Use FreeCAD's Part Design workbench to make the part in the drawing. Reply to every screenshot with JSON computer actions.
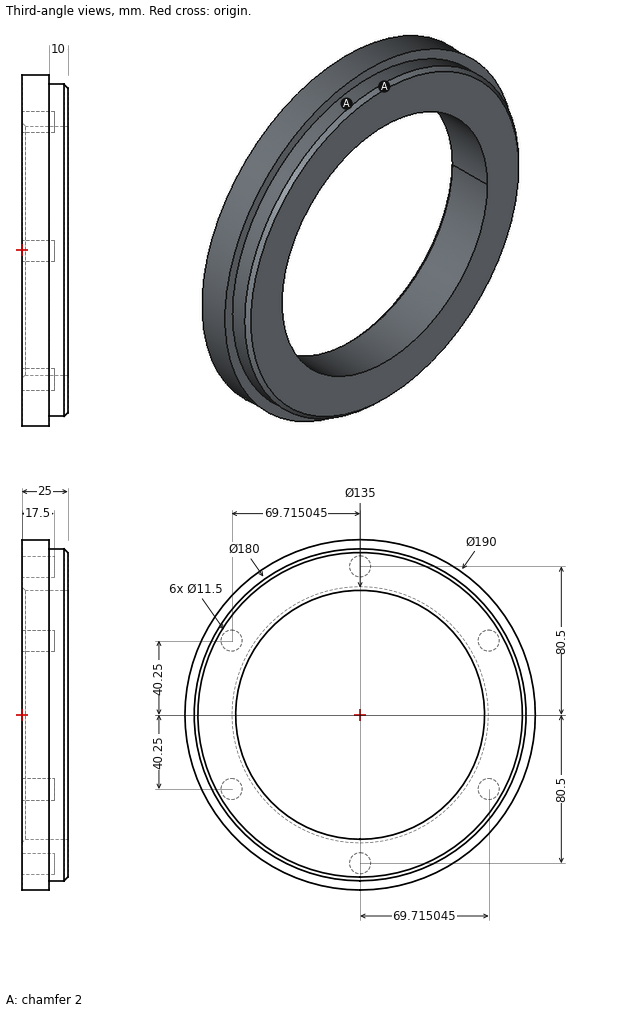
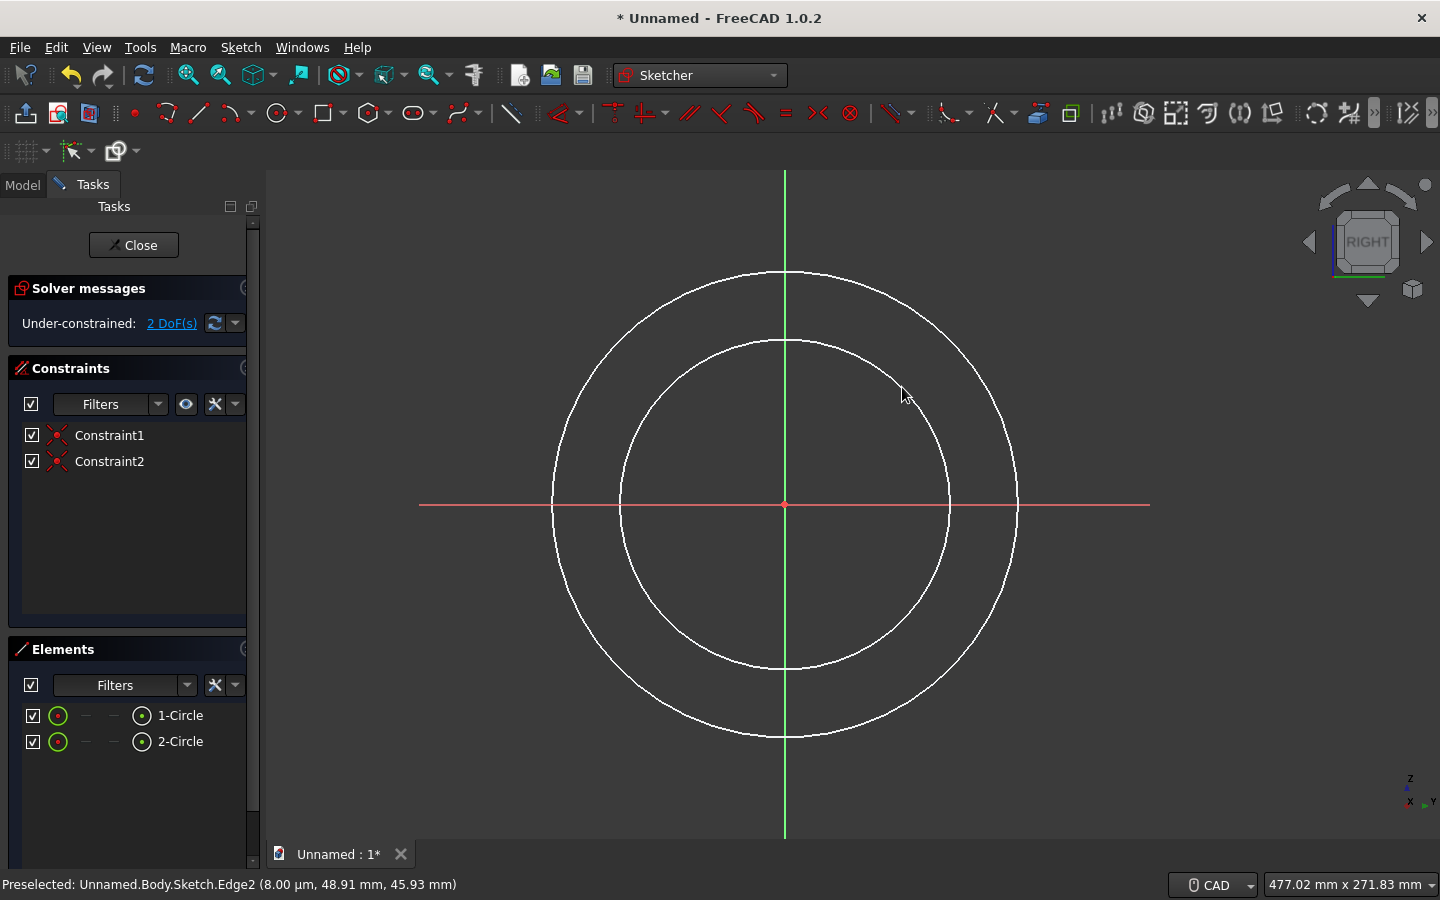
{"action": "left_click", "coordinate": [558, 114]}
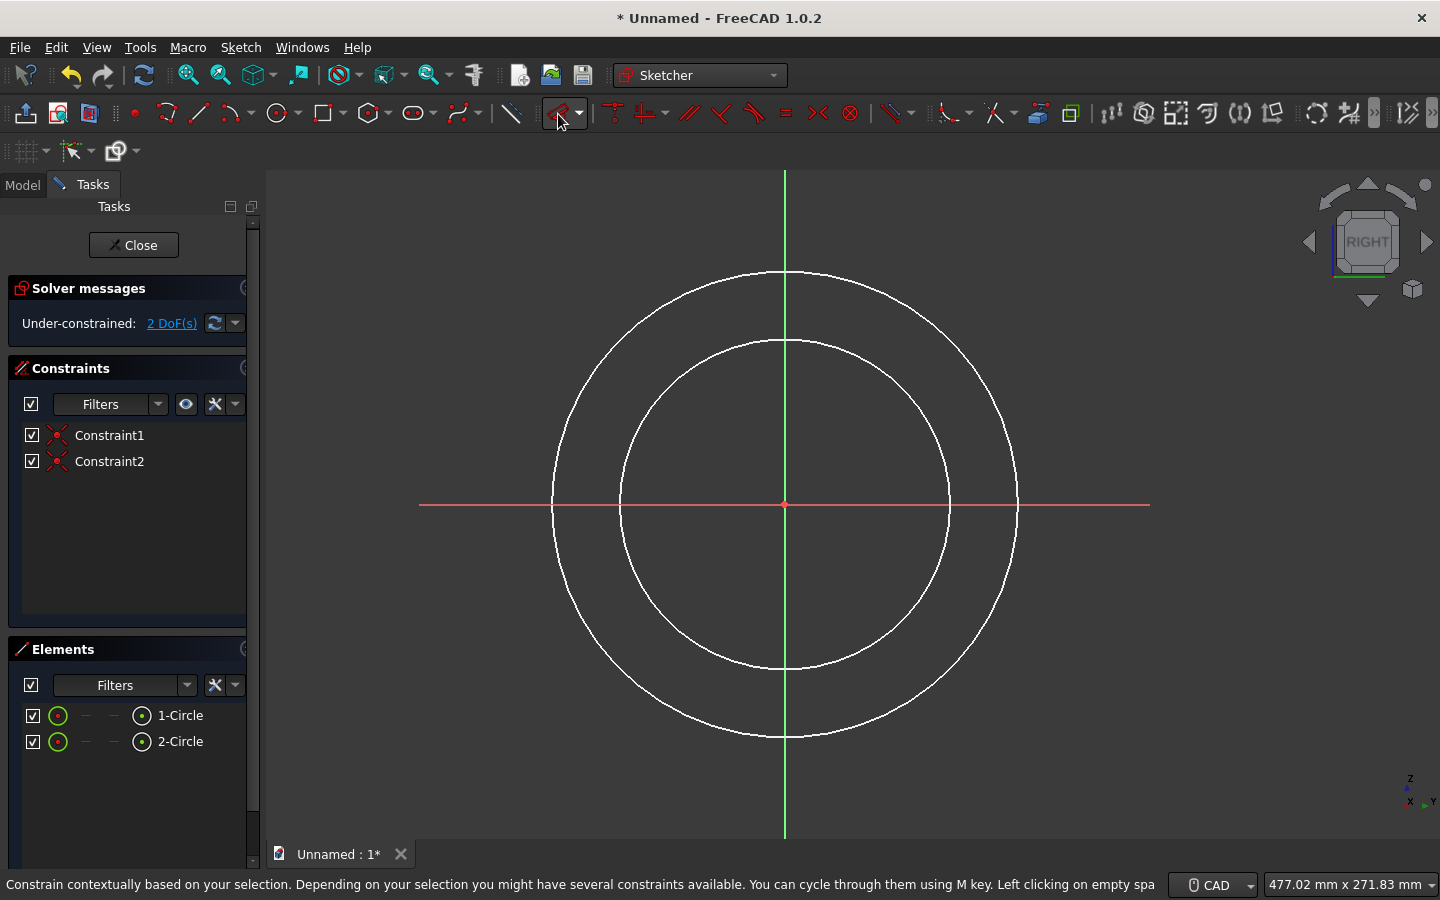
{"action": "left_click", "coordinate": [949, 339]}
{"action": "left_click", "coordinate": [972, 316]}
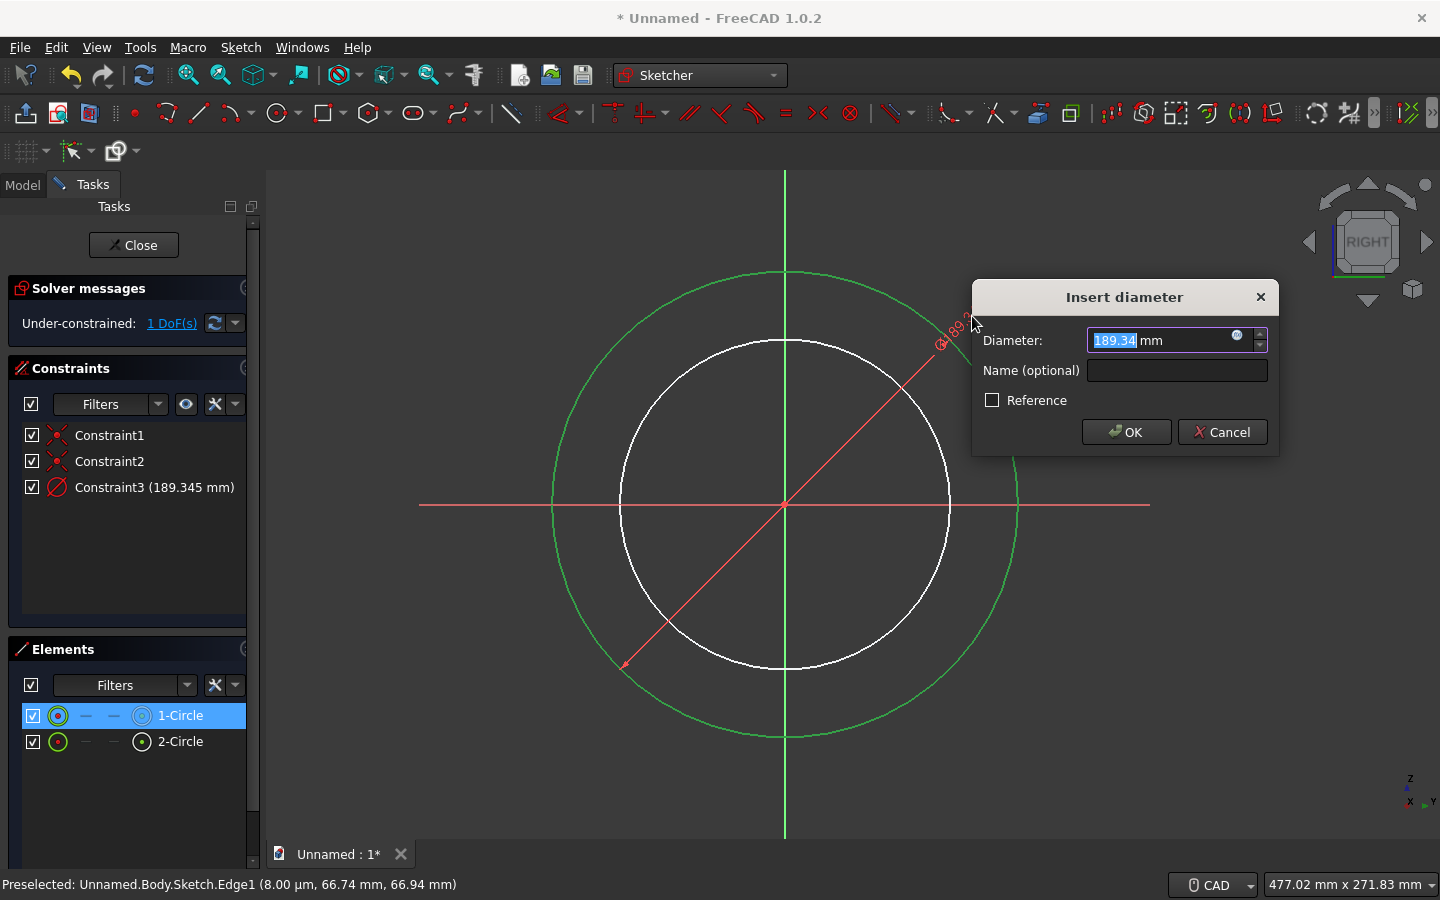
{"action": "type", "text": "190"}
{"action": "key", "text": "Return"}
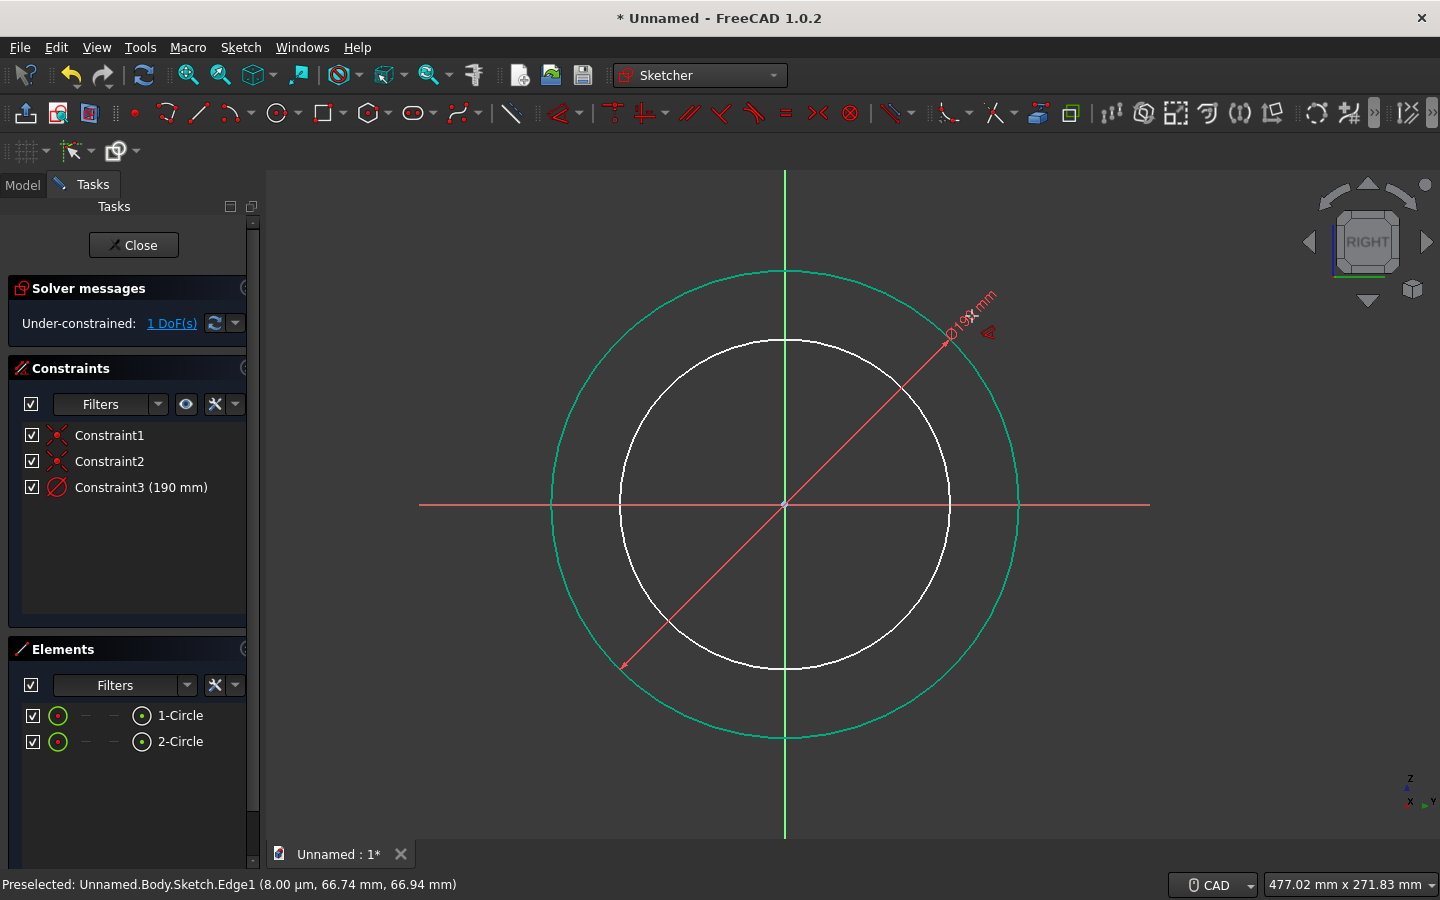
{"action": "left_click", "coordinate": [901, 387]}
{"action": "left_click", "coordinate": [923, 364]}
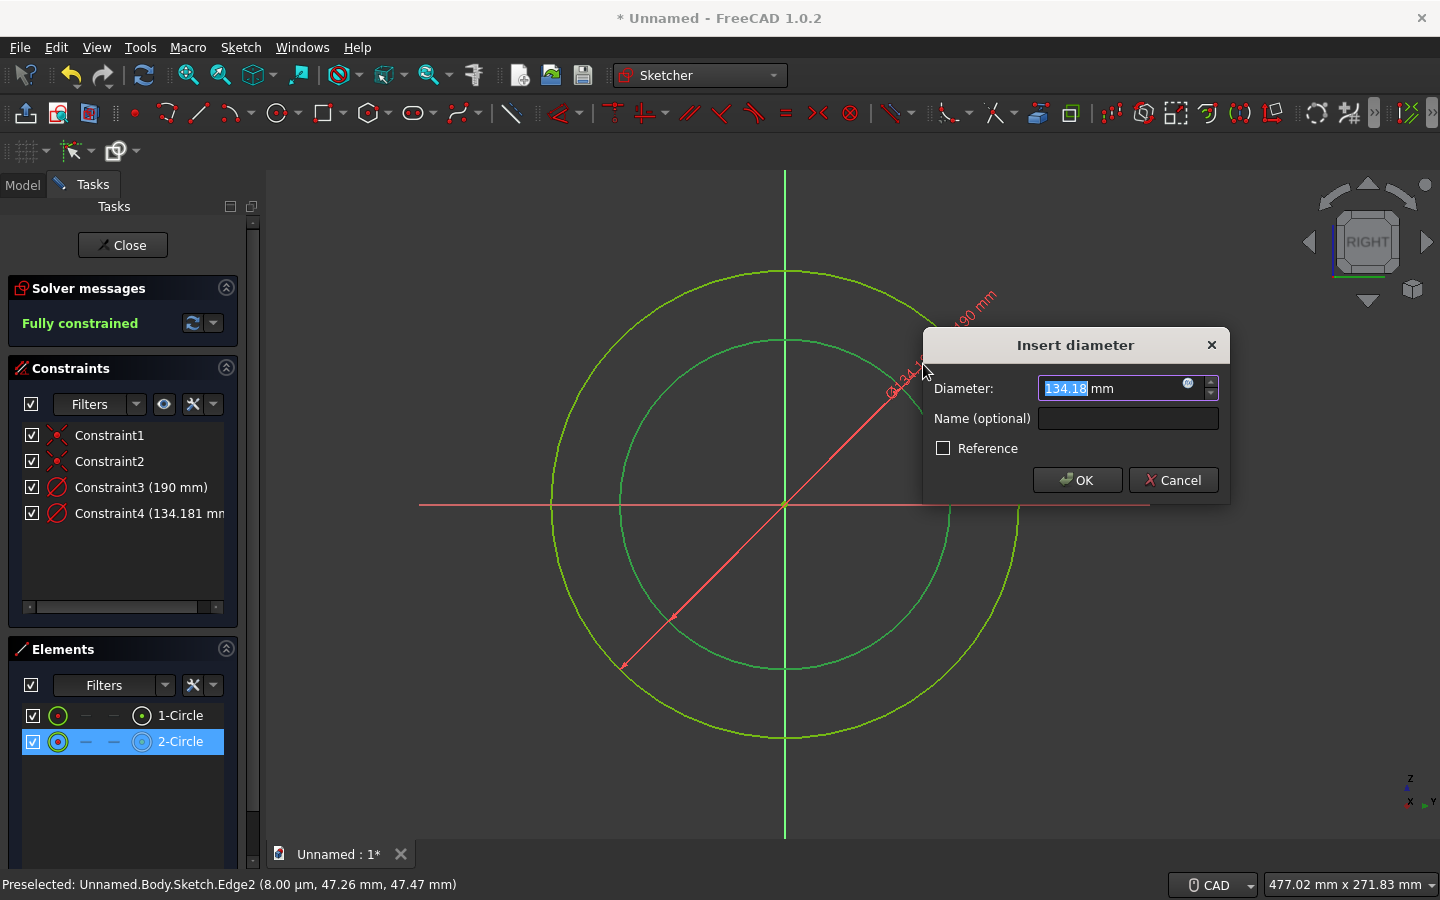
{"action": "type", "text": "135"}
{"action": "key", "text": "Return"}
{"action": "key", "text": "Escape"}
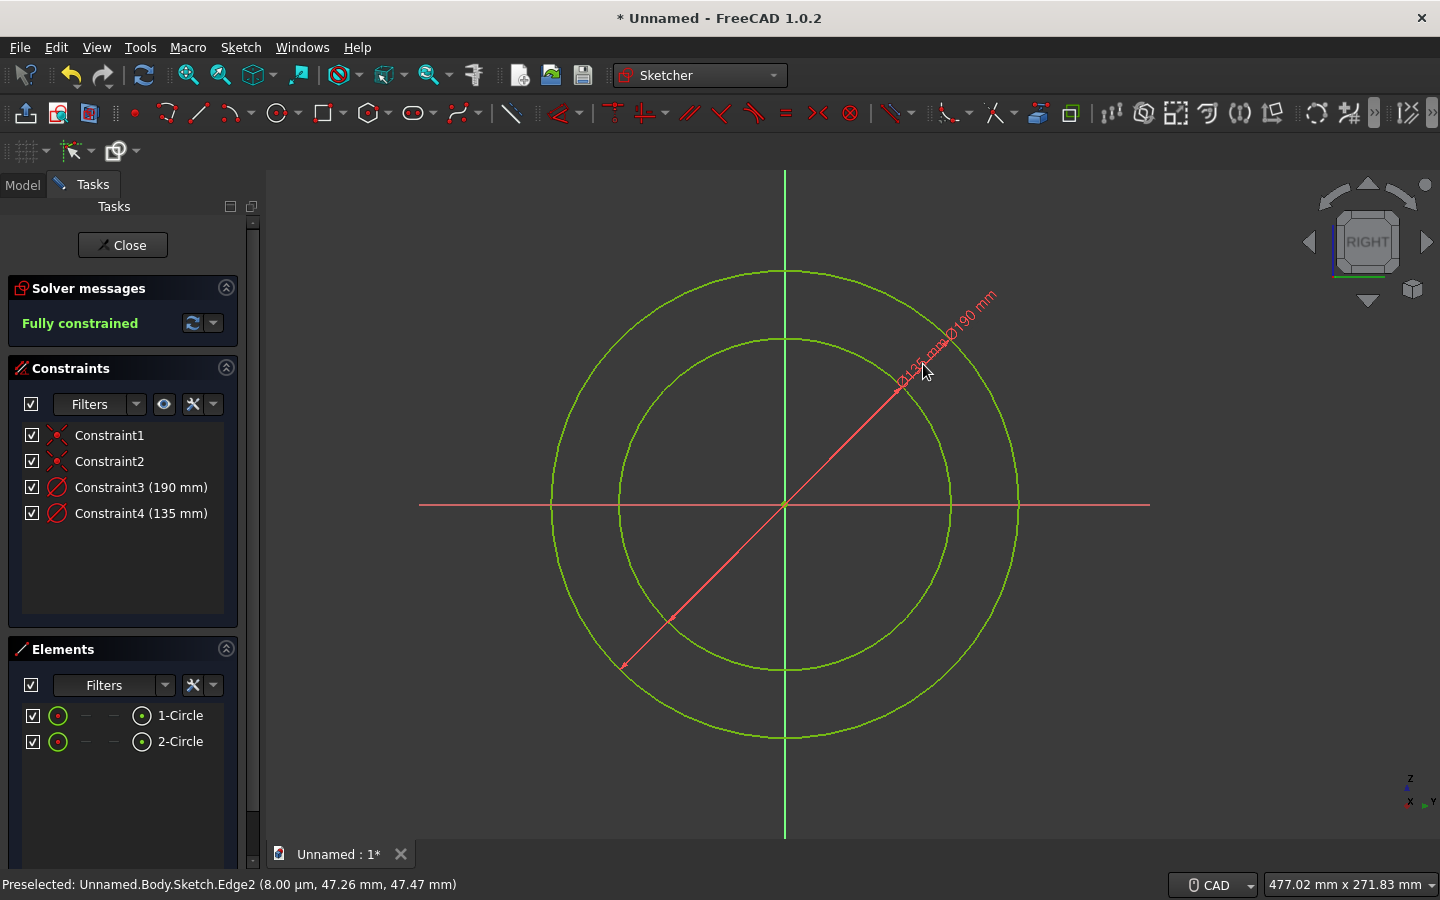
{"action": "left_click", "coordinate": [123, 245]}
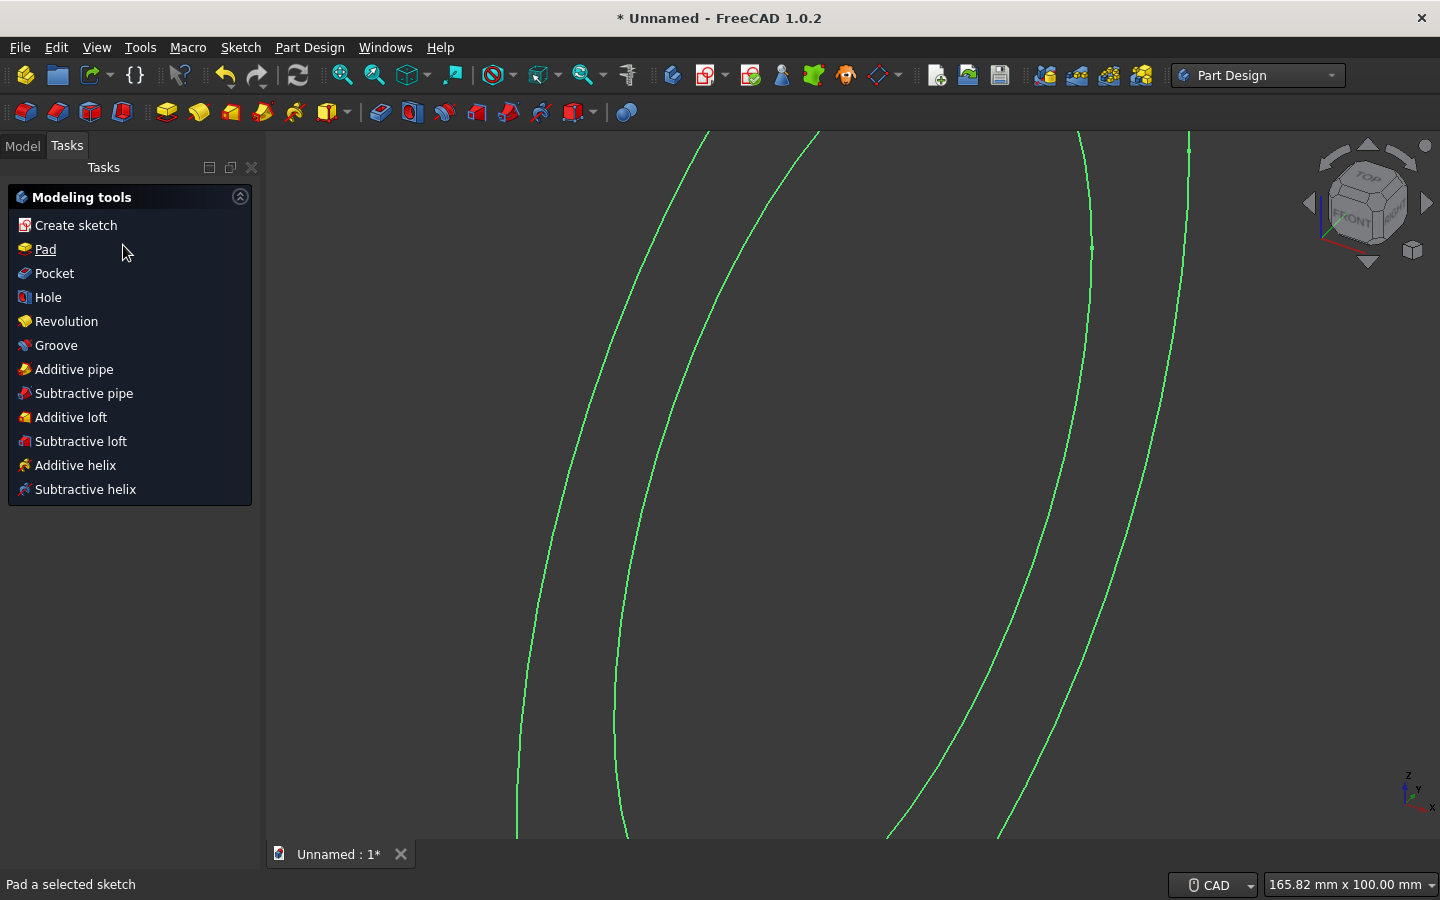
{"action": "left_click", "coordinate": [168, 112]}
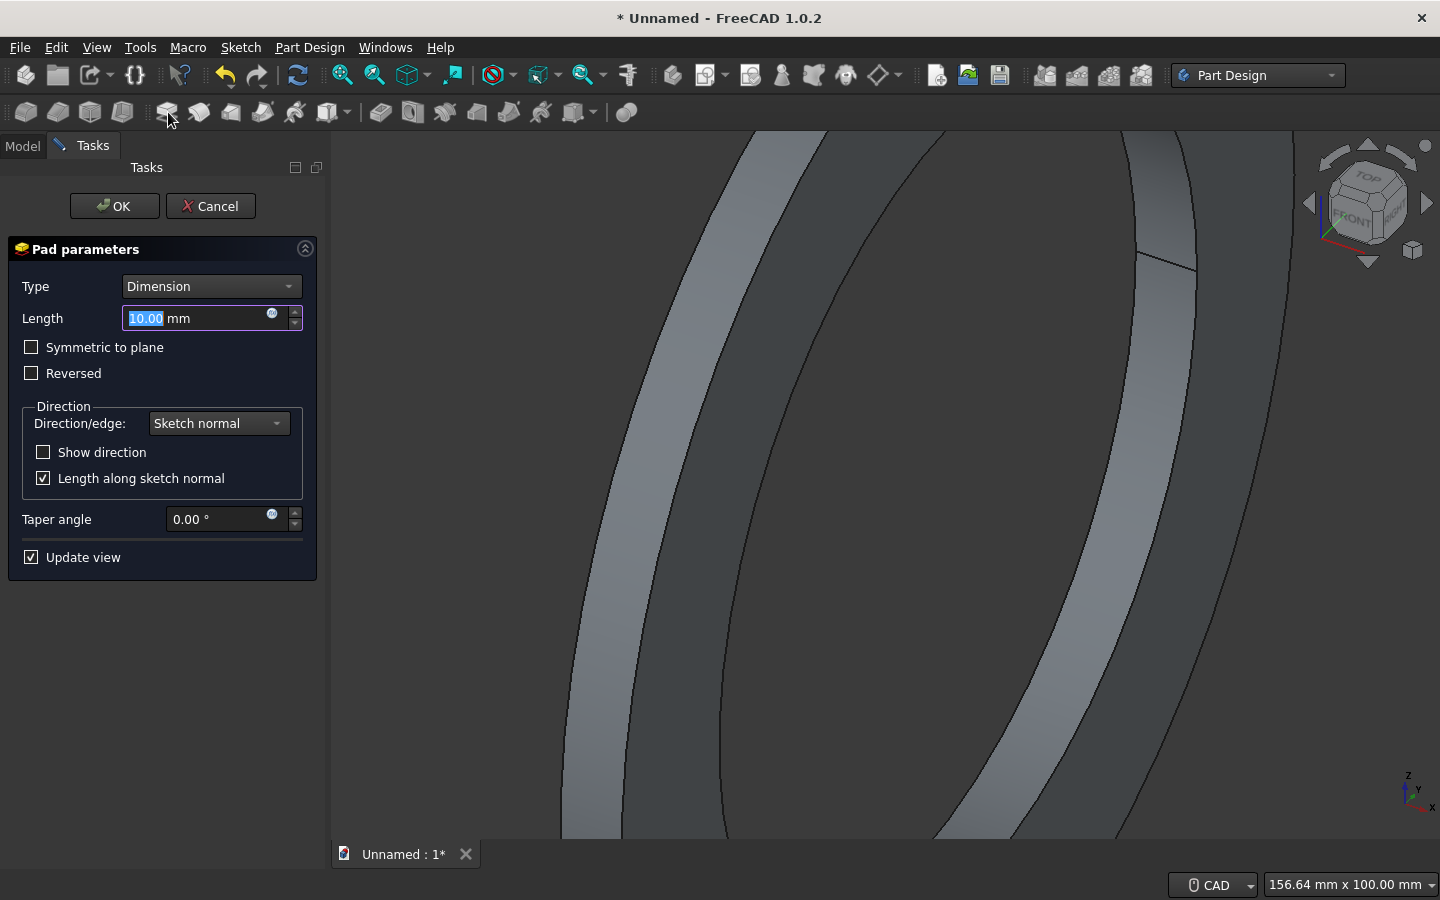
{"action": "type", "text": "25"}
{"action": "key", "text": "Tab"}